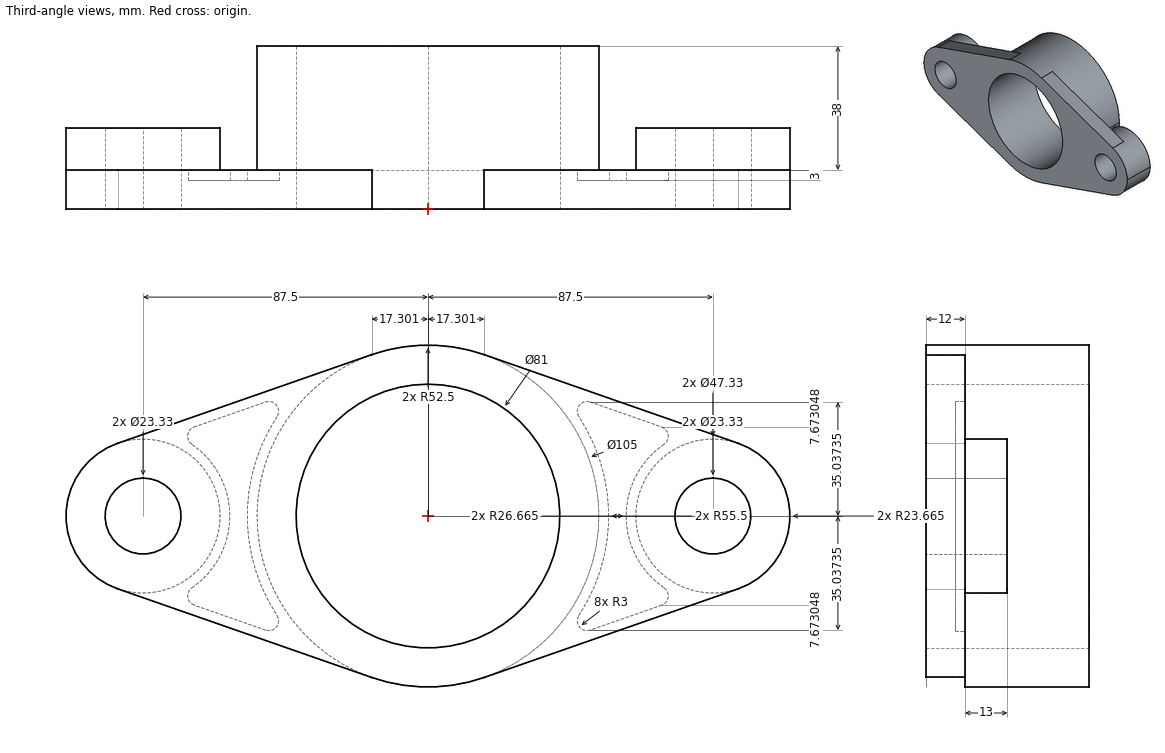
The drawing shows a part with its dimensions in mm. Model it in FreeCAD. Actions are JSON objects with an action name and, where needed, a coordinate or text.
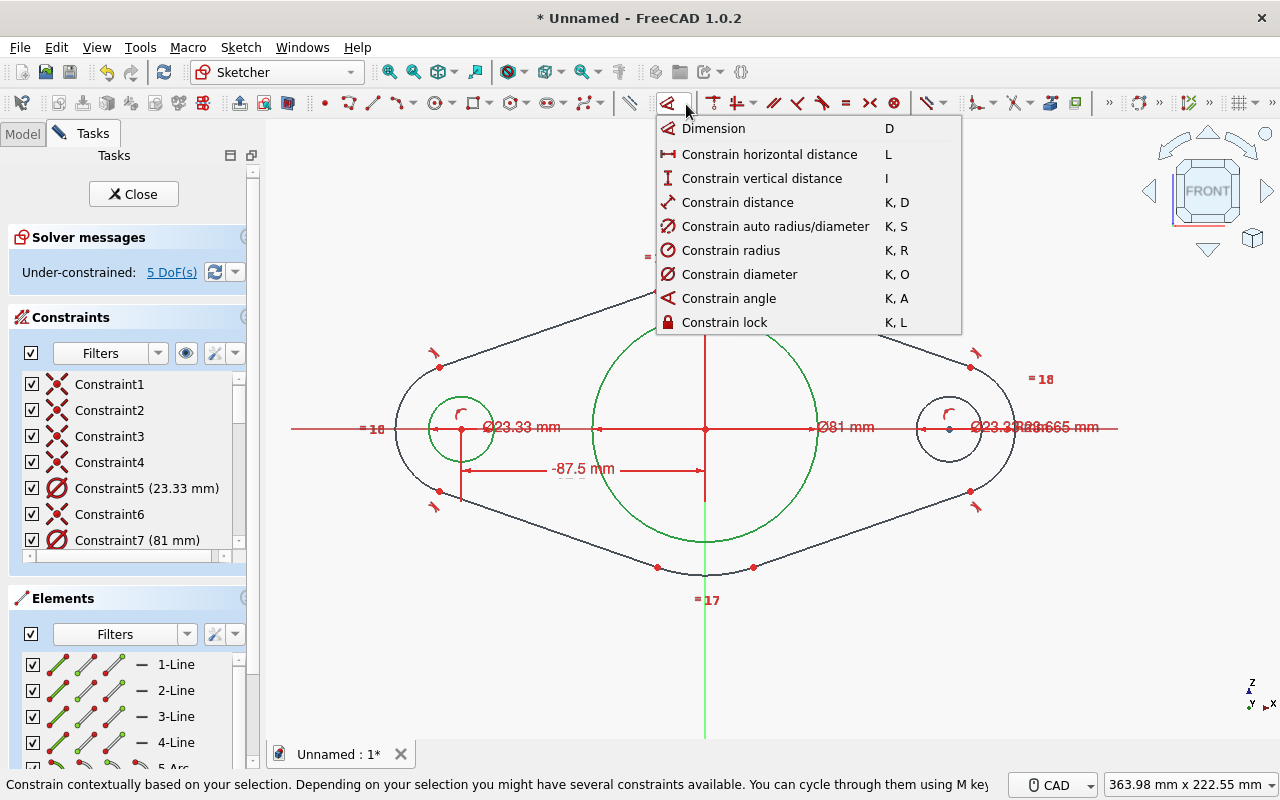
{"action": "left_click", "coordinate": [809, 154]}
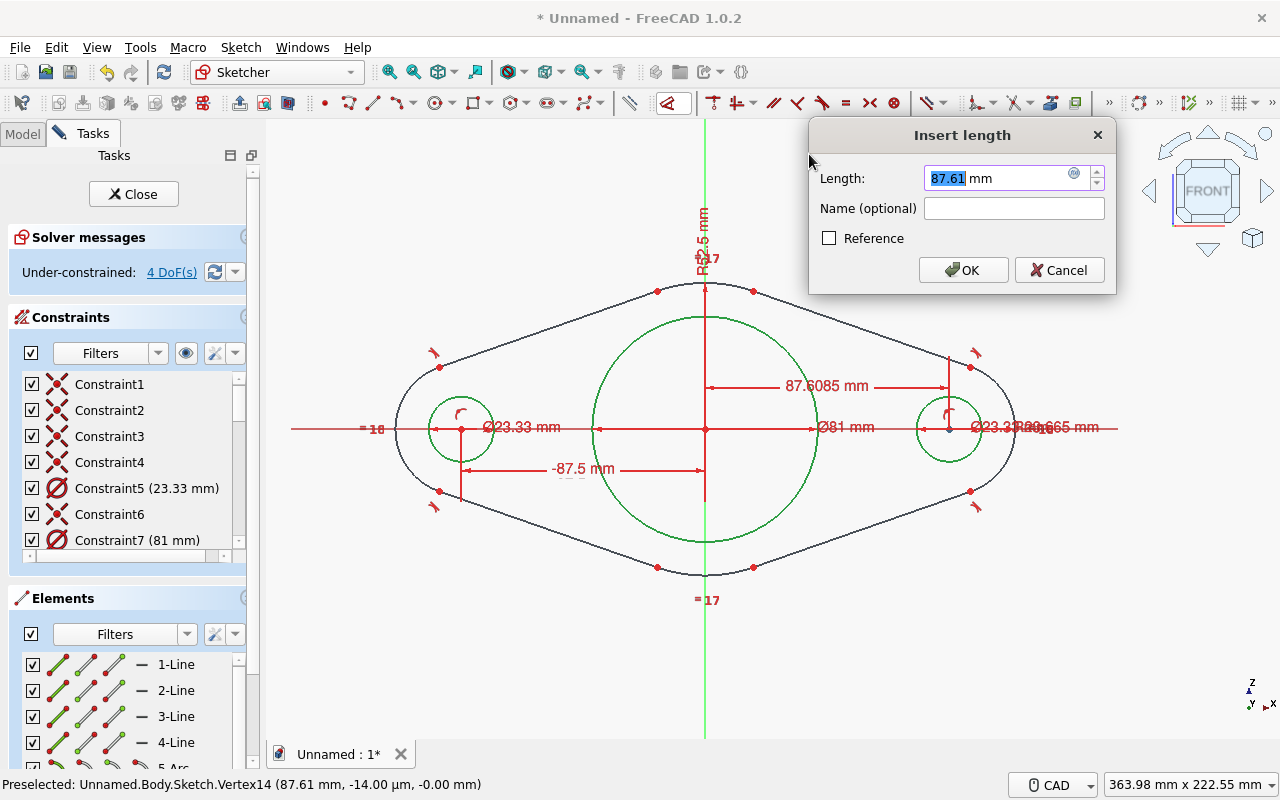
{"action": "type", "text": "87.5"}
{"action": "key", "text": "Return"}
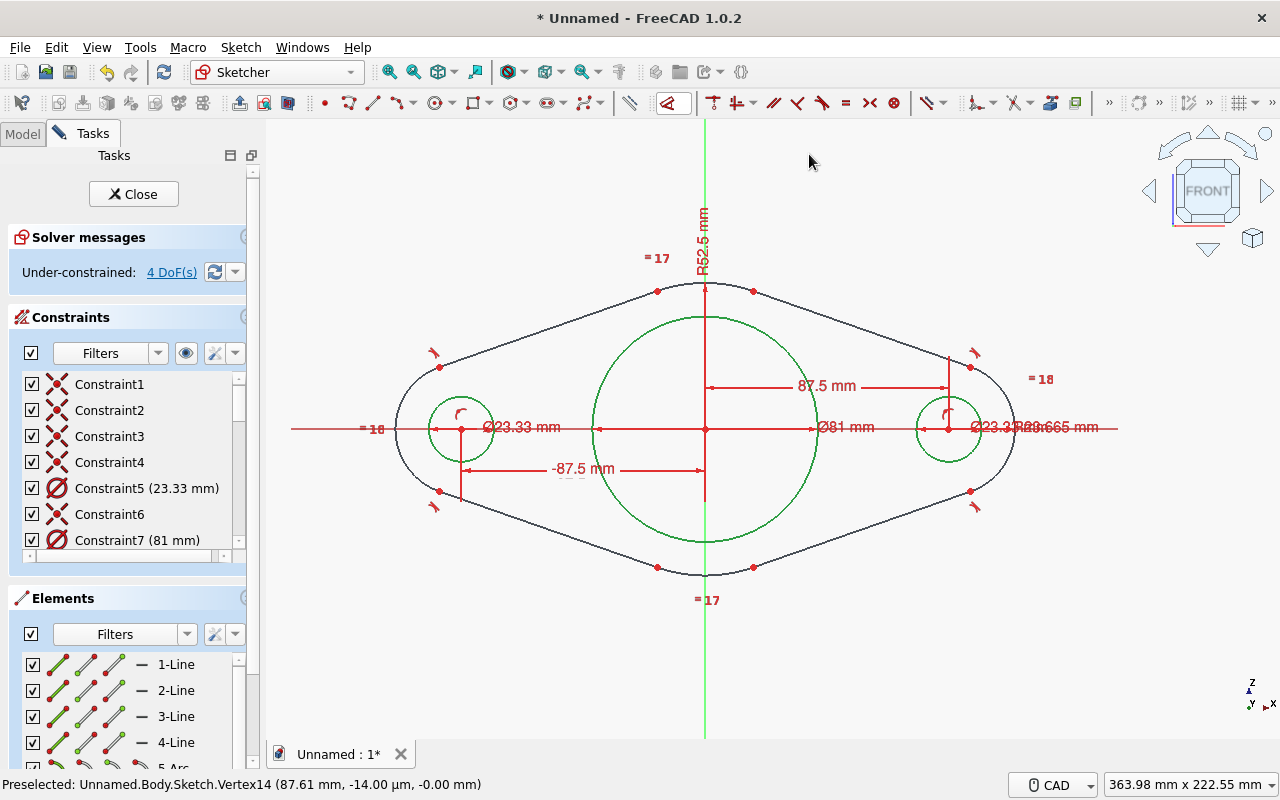
{"action": "left_click", "coordinate": [657, 291]}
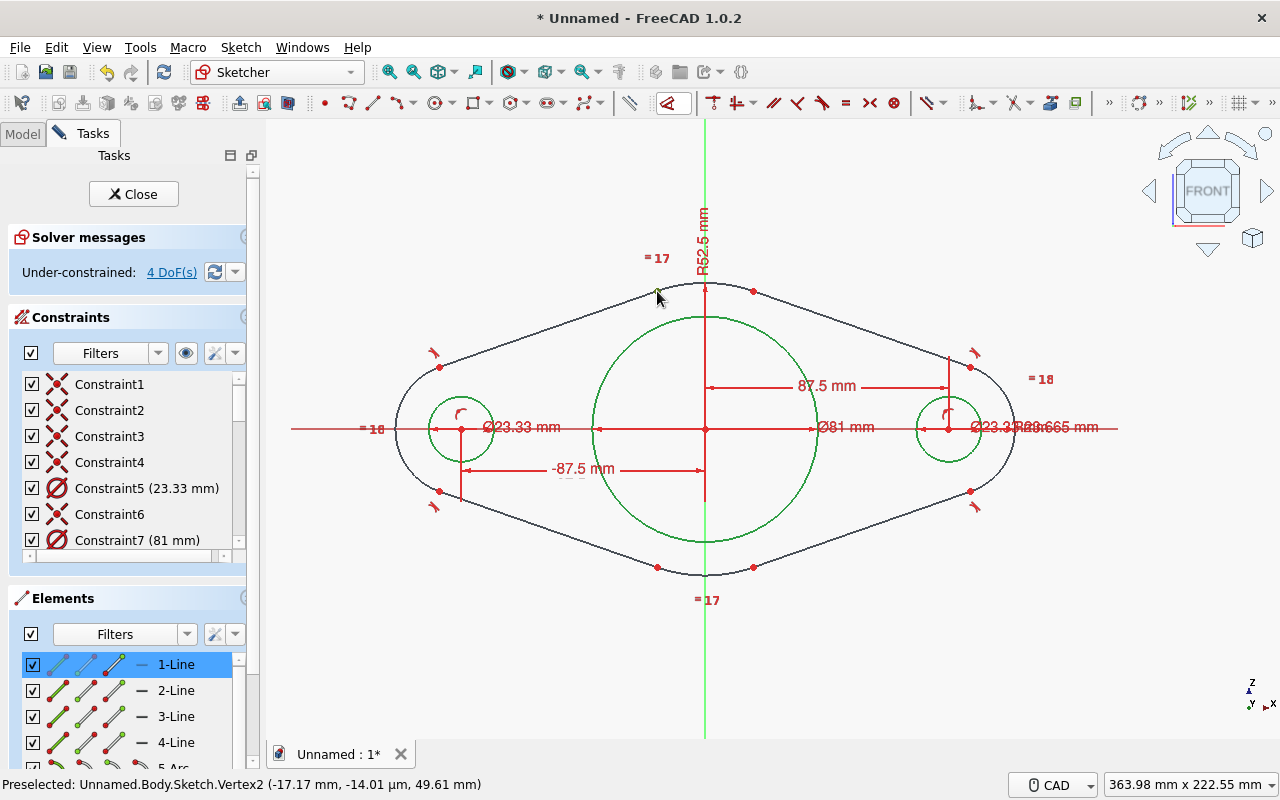
{"action": "key", "text": "l"}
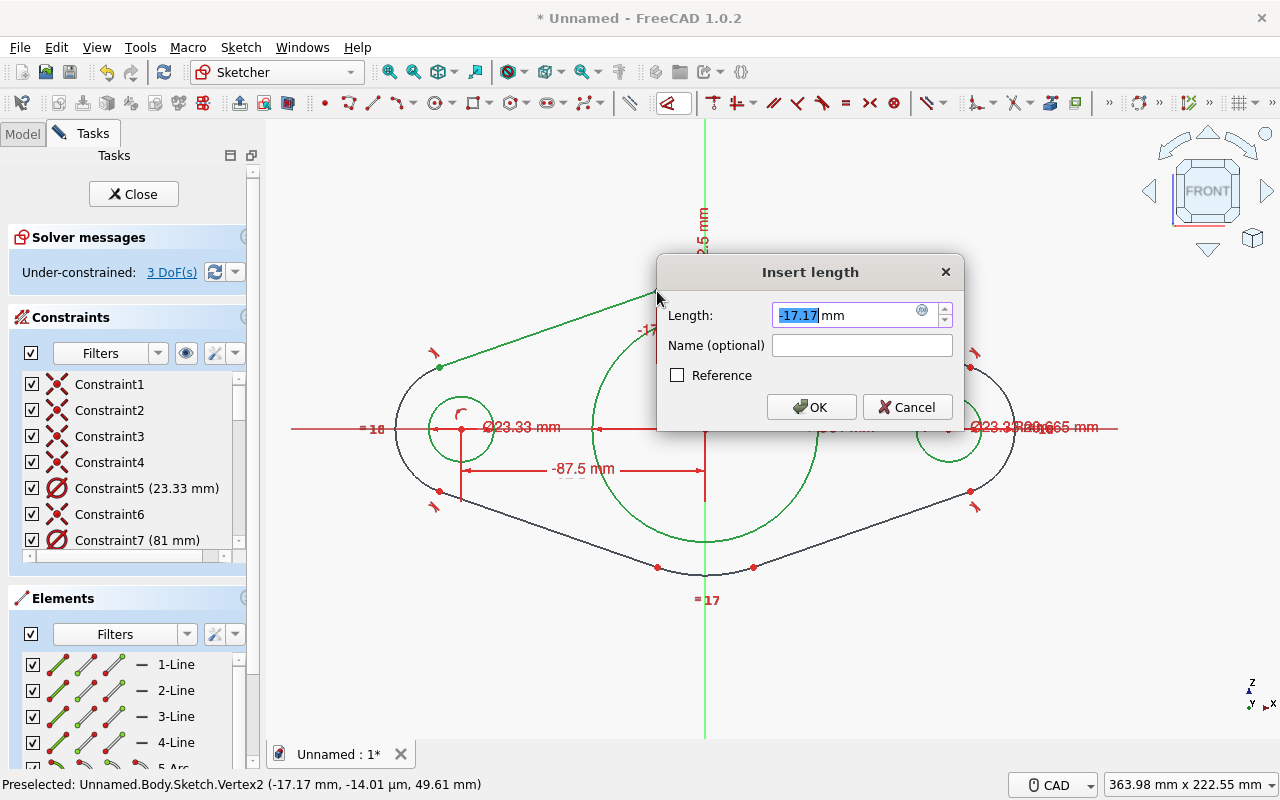
{"action": "type", "text": "-17.301"}
{"action": "key", "text": "Return"}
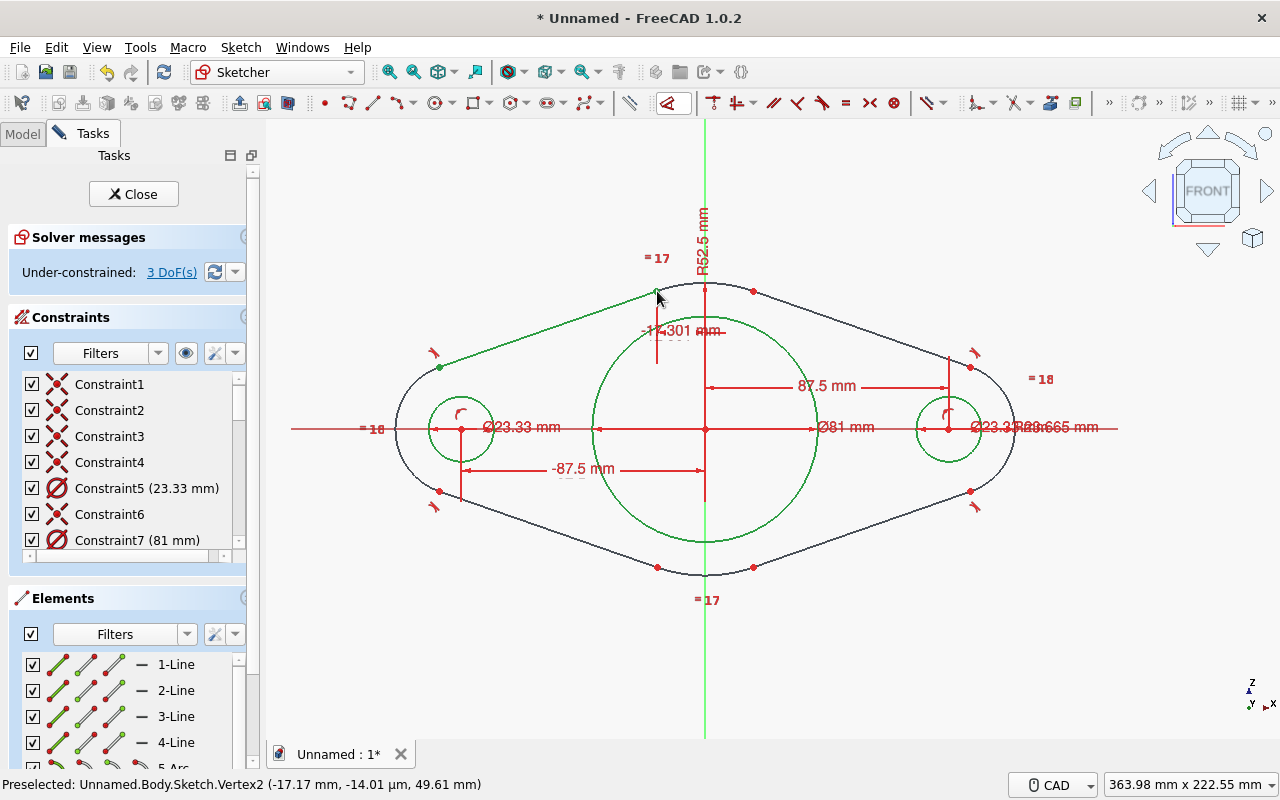
{"action": "left_click", "coordinate": [753, 291]}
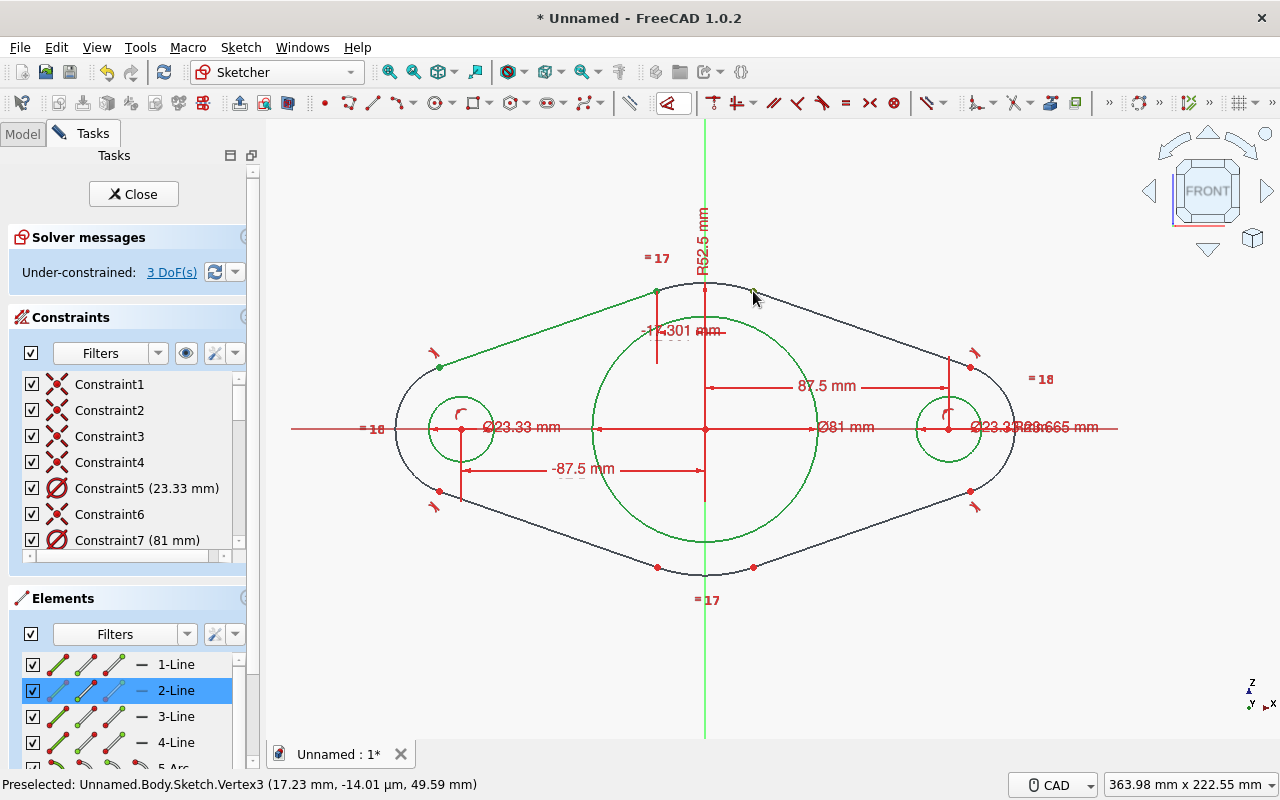
{"action": "key", "text": "l"}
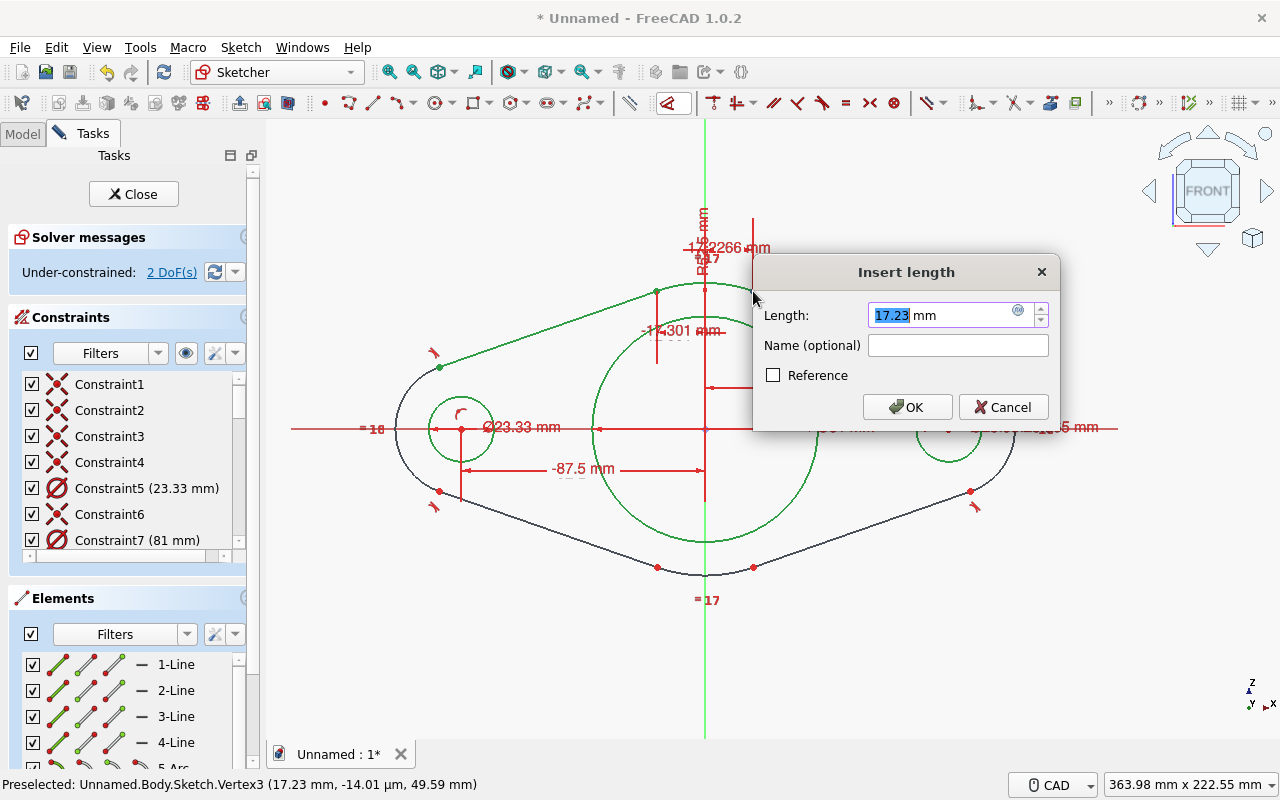
{"action": "type", "text": "17.301"}
{"action": "key", "text": "Return"}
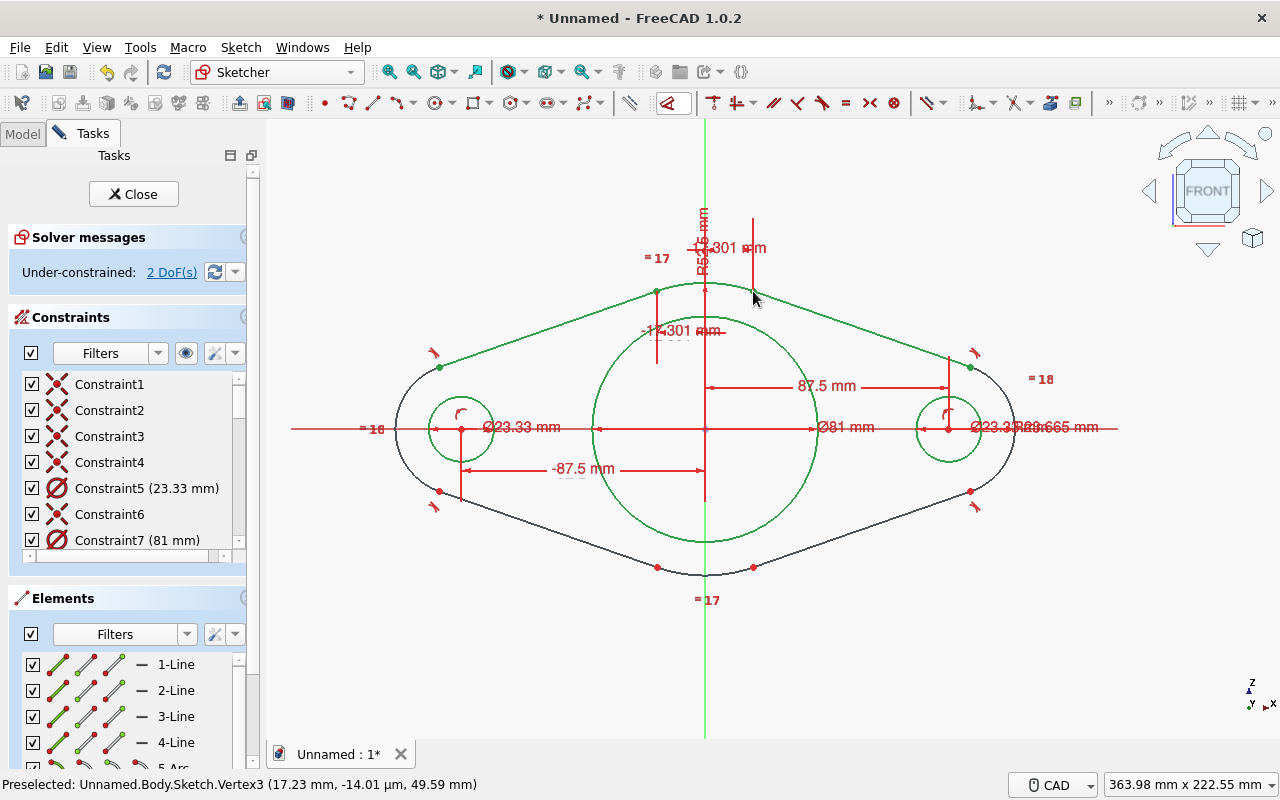
{"action": "left_click", "coordinate": [753, 567]}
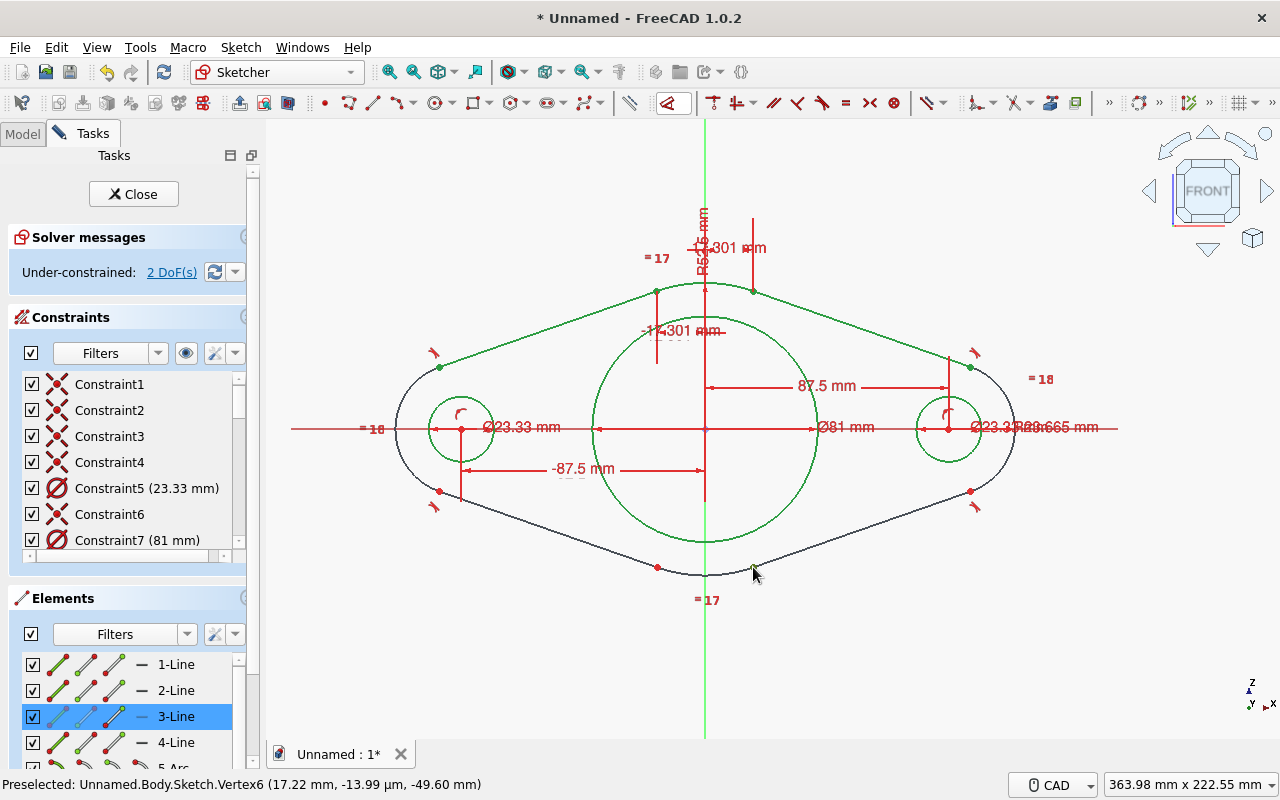
{"action": "key", "text": "l"}